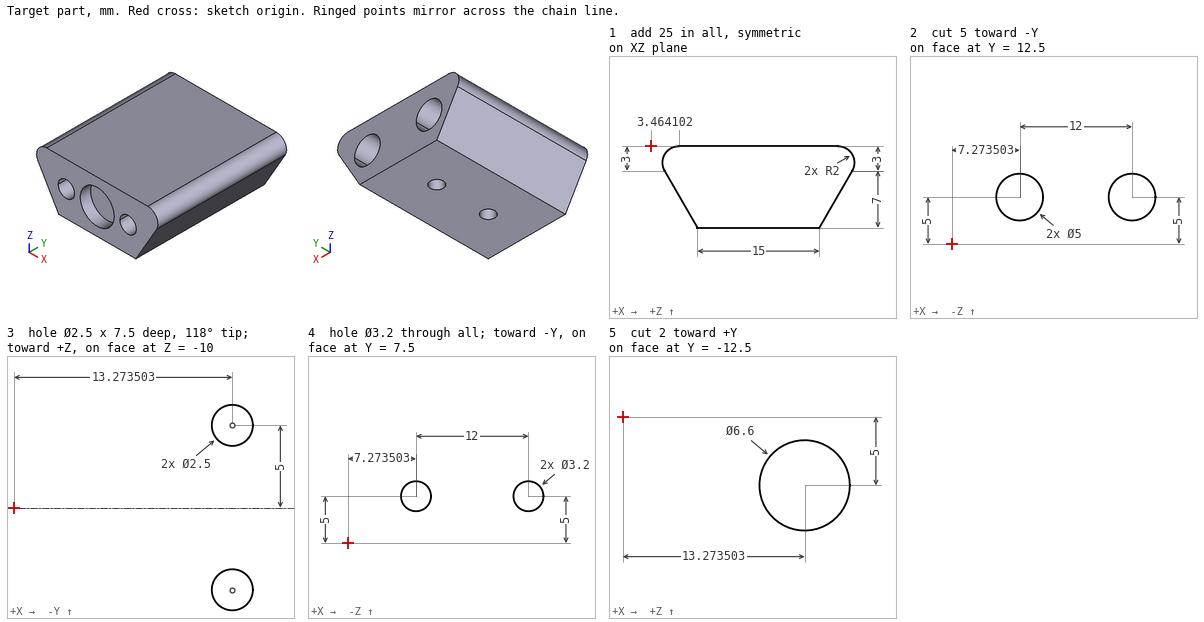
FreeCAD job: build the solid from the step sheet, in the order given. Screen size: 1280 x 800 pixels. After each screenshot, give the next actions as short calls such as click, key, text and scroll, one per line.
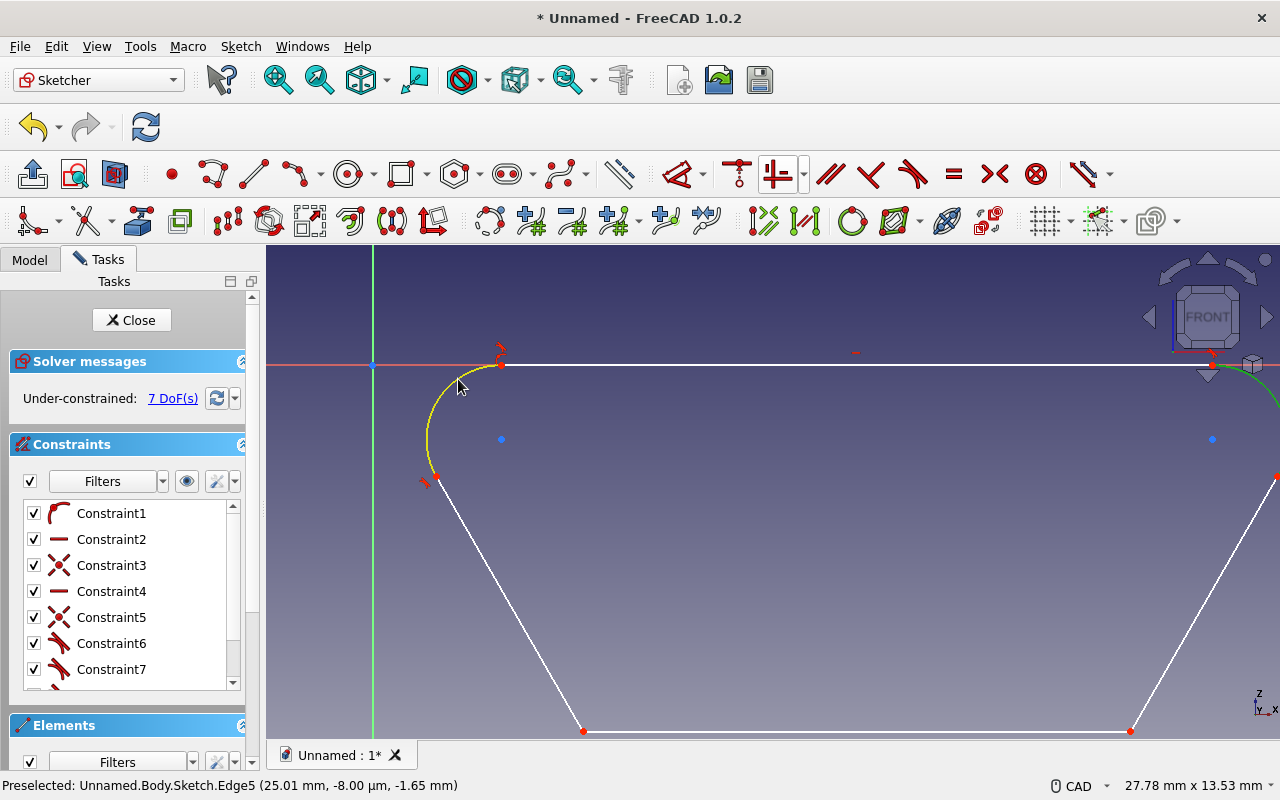
click(457, 379)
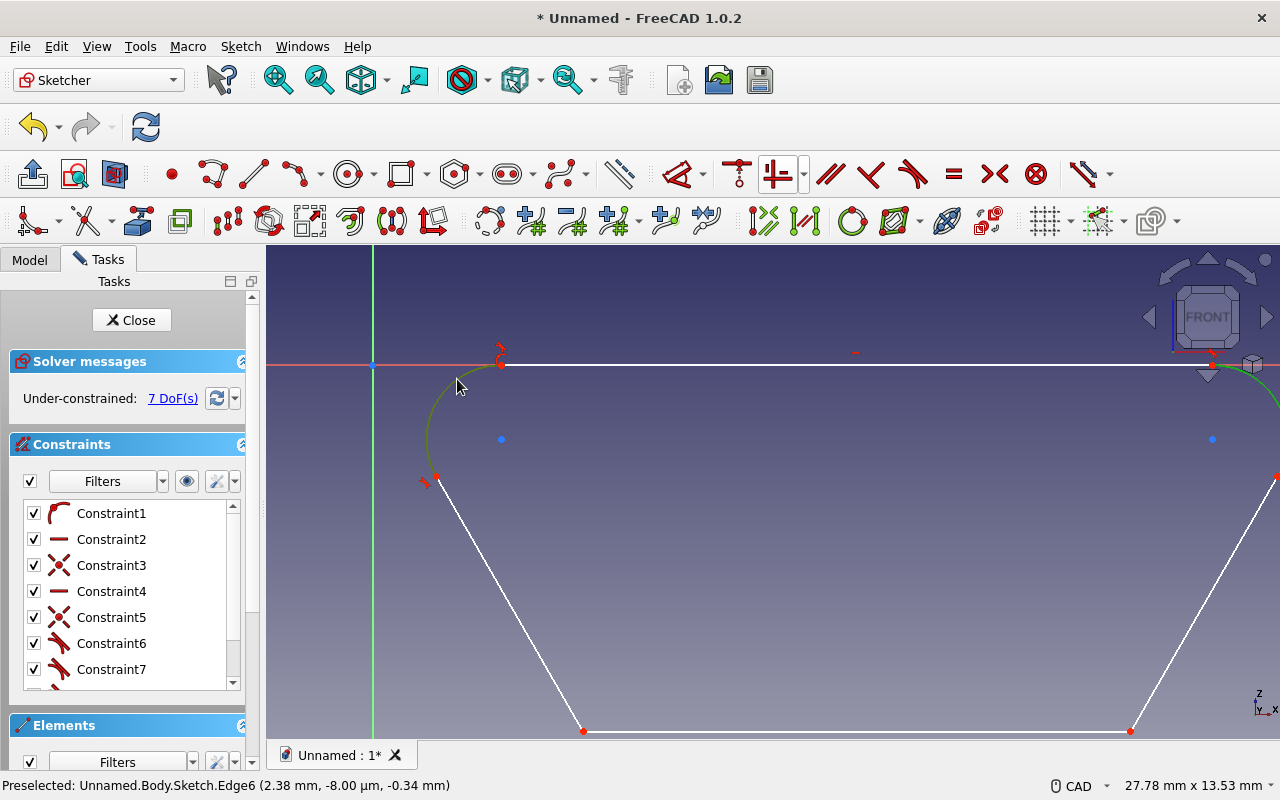
click(954, 174)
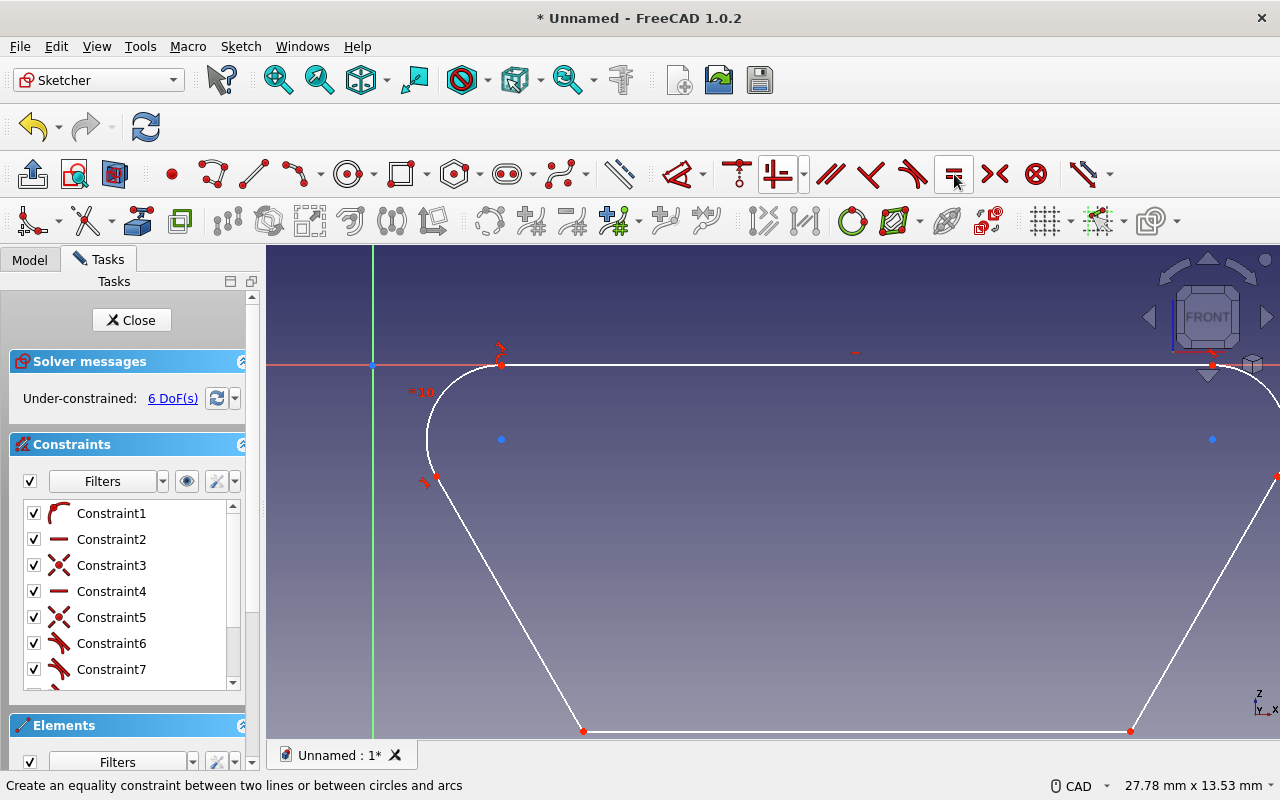
click(676, 174)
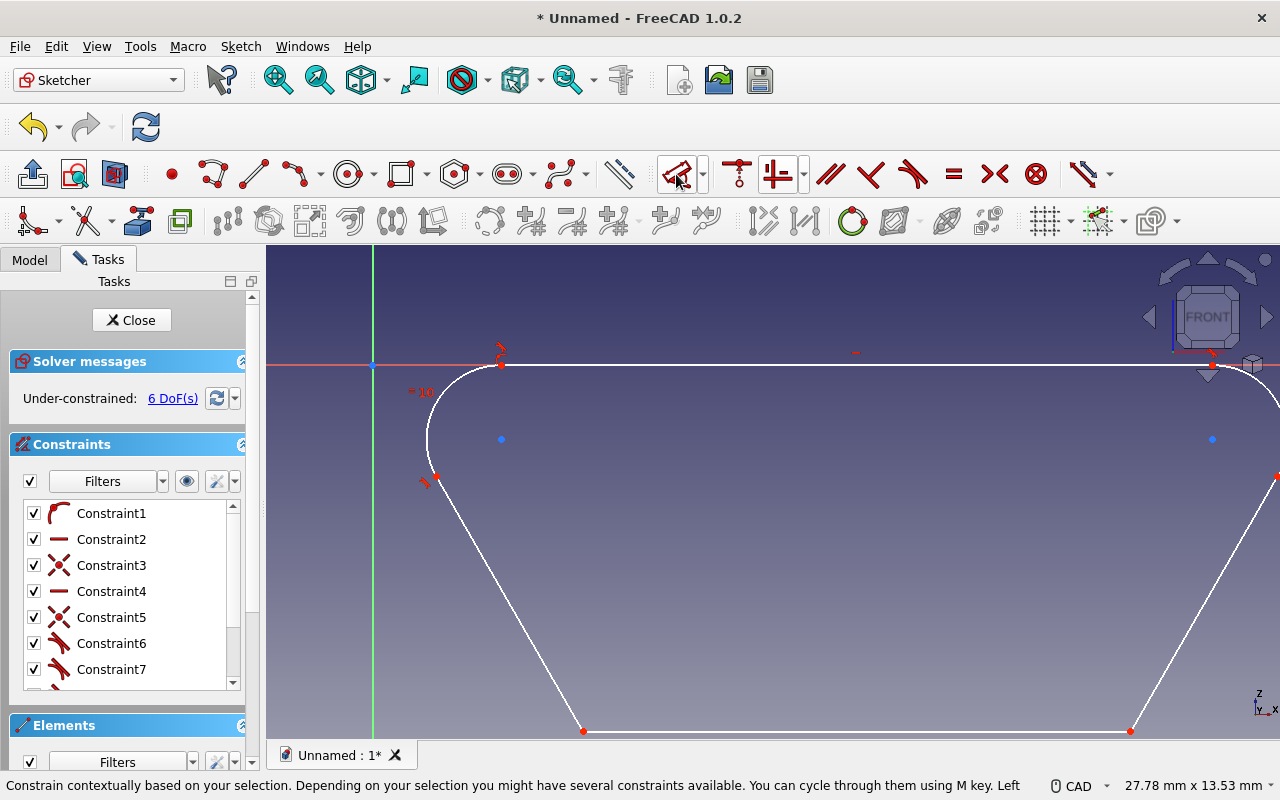
scroll(458, 379, down, 2)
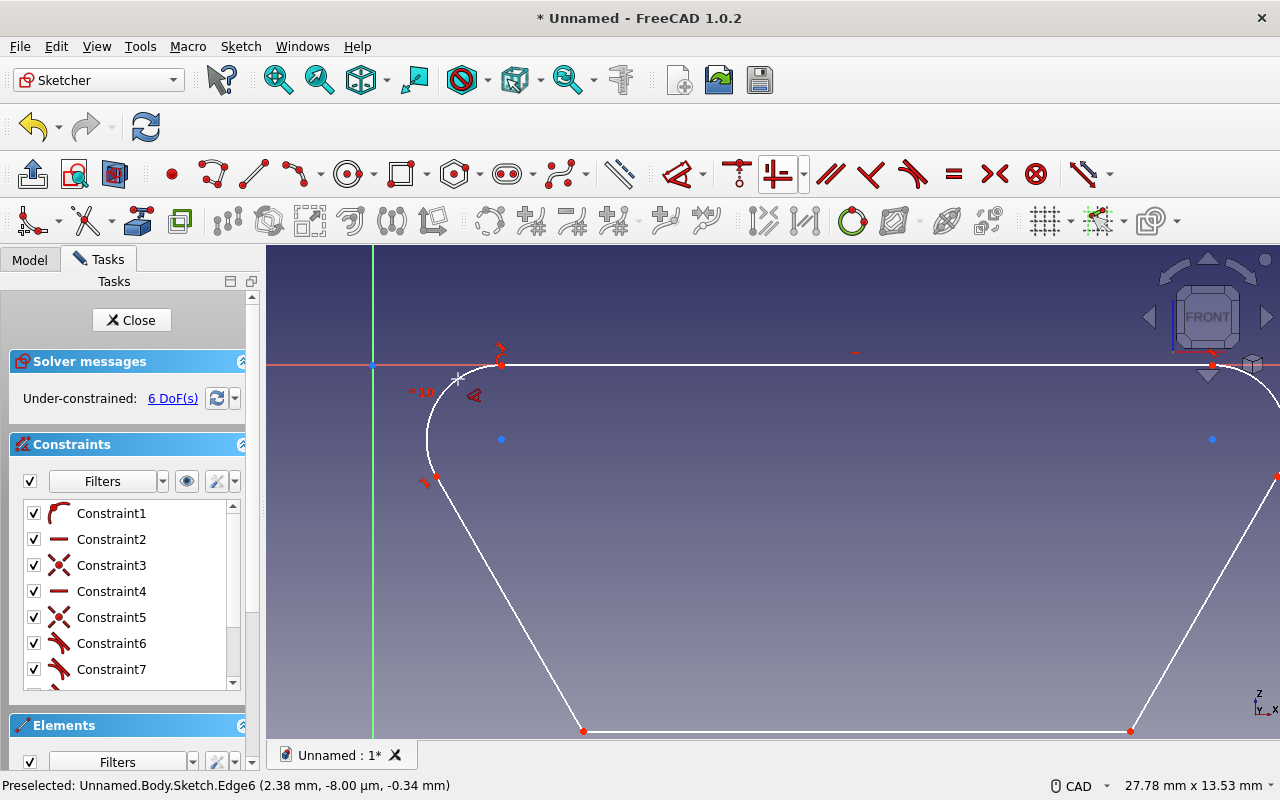
click(1014, 414)
click(1046, 410)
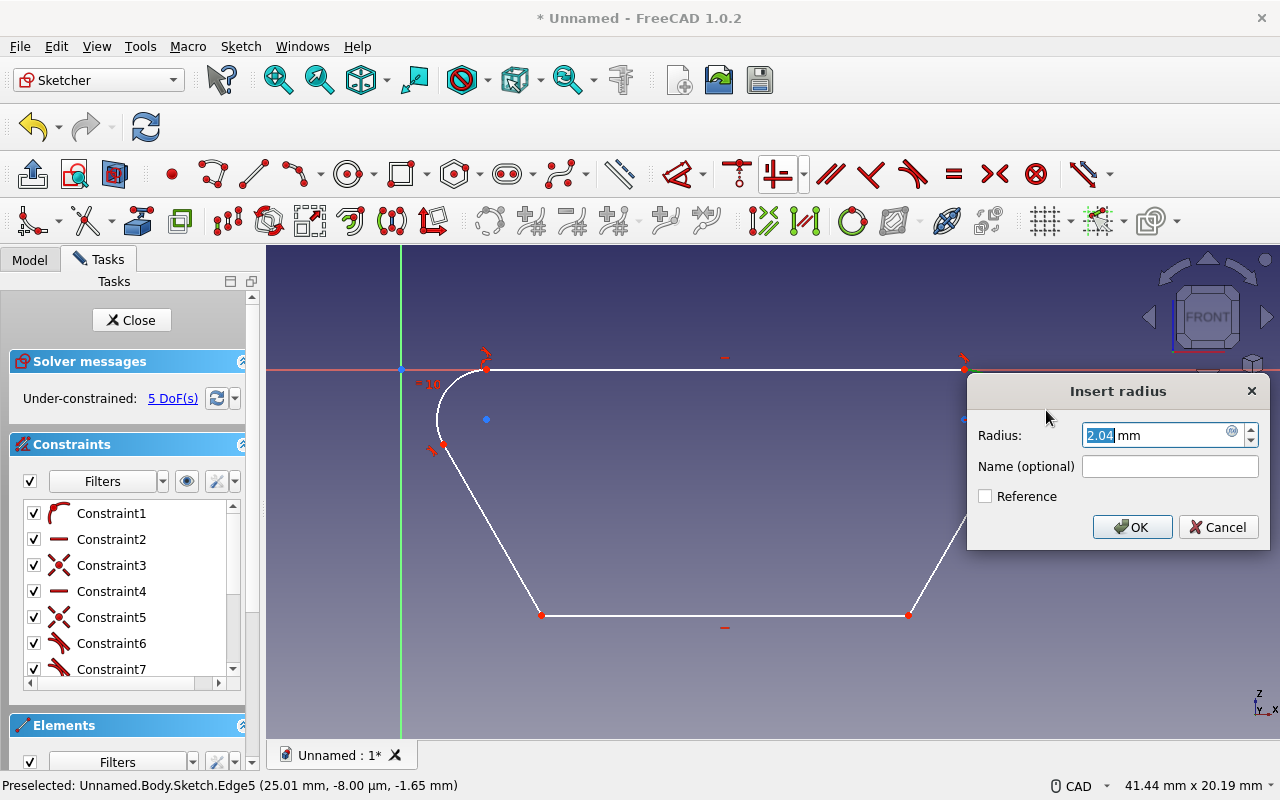
text(2)
key(Return)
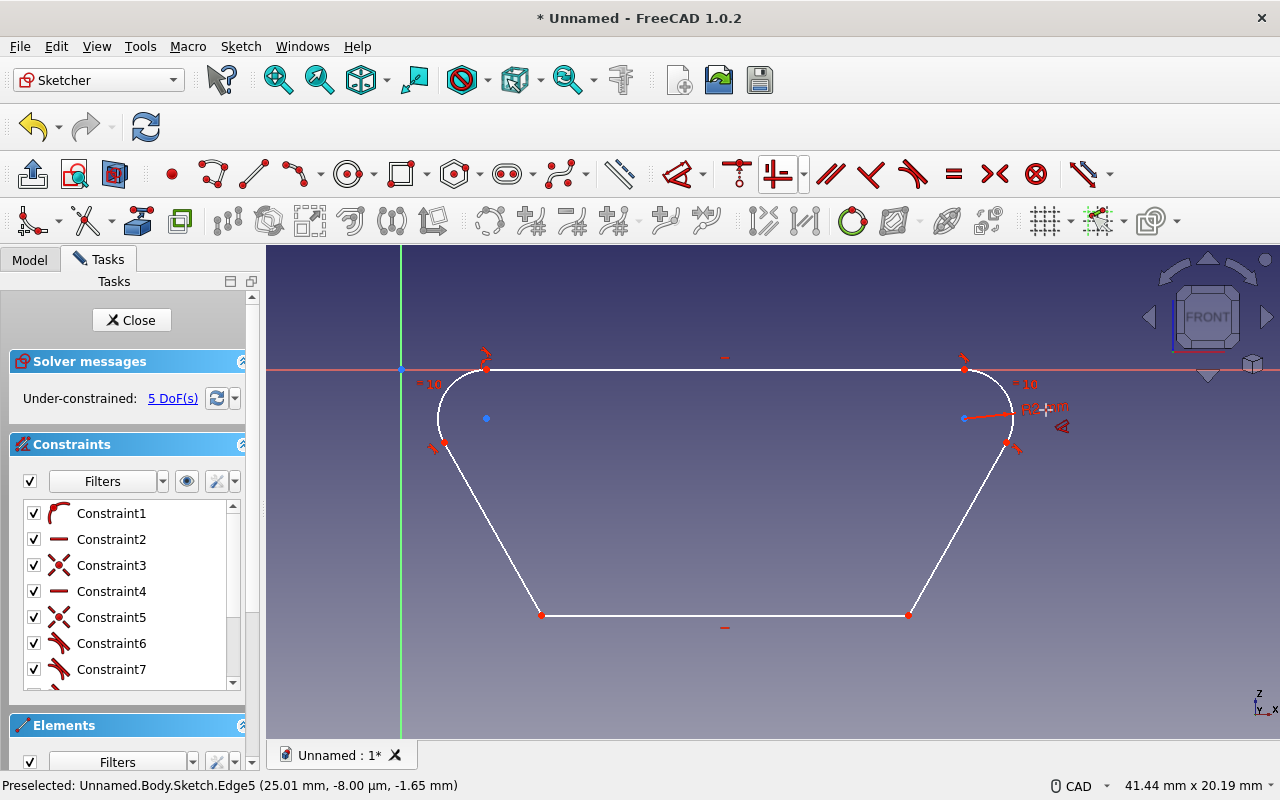
click(799, 616)
click(725, 650)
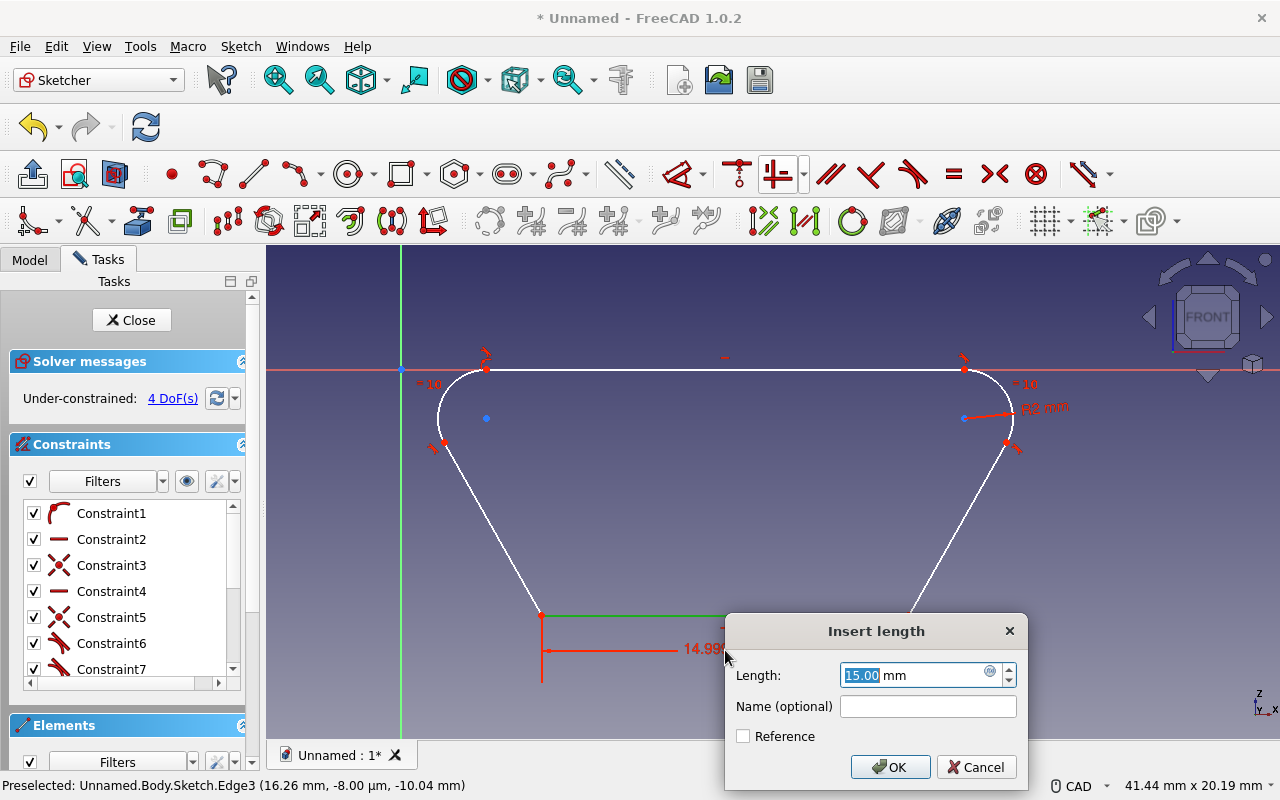
text(15)
key(Return)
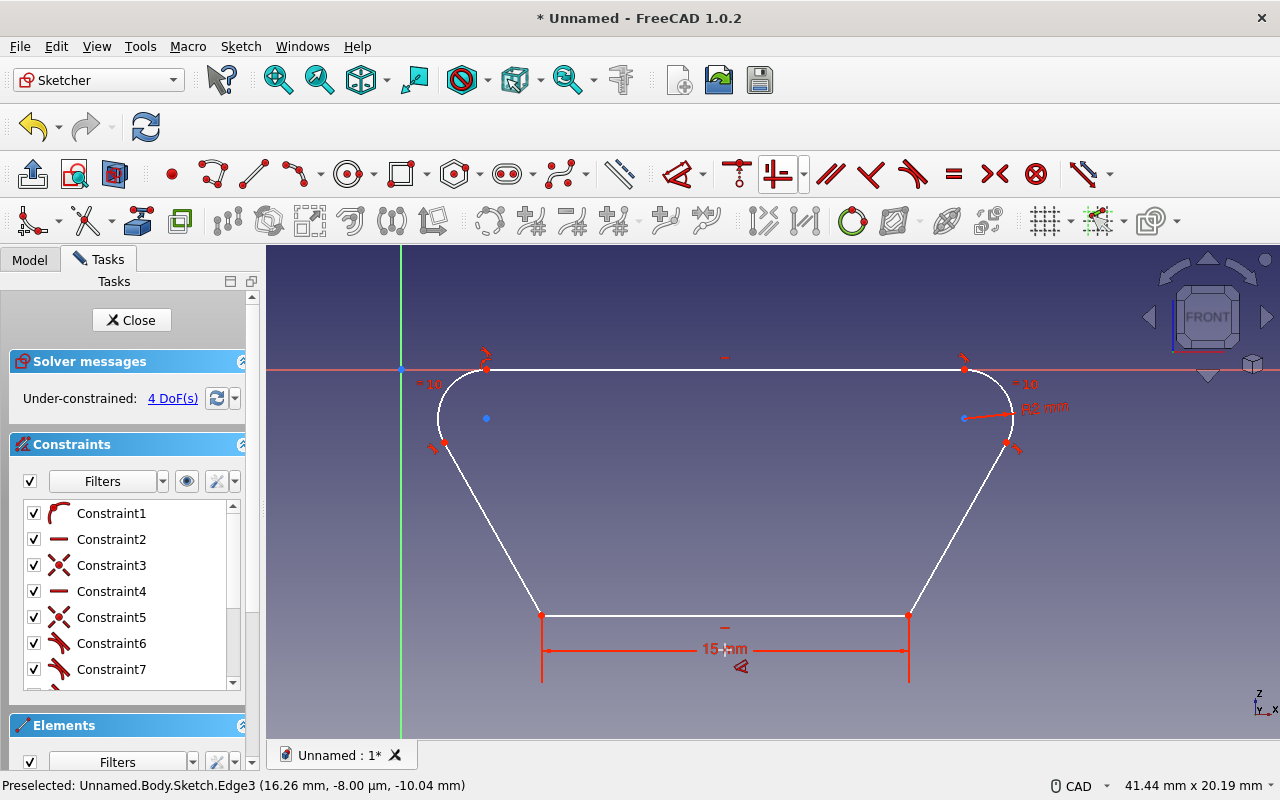
click(1007, 443)
click(367, 406)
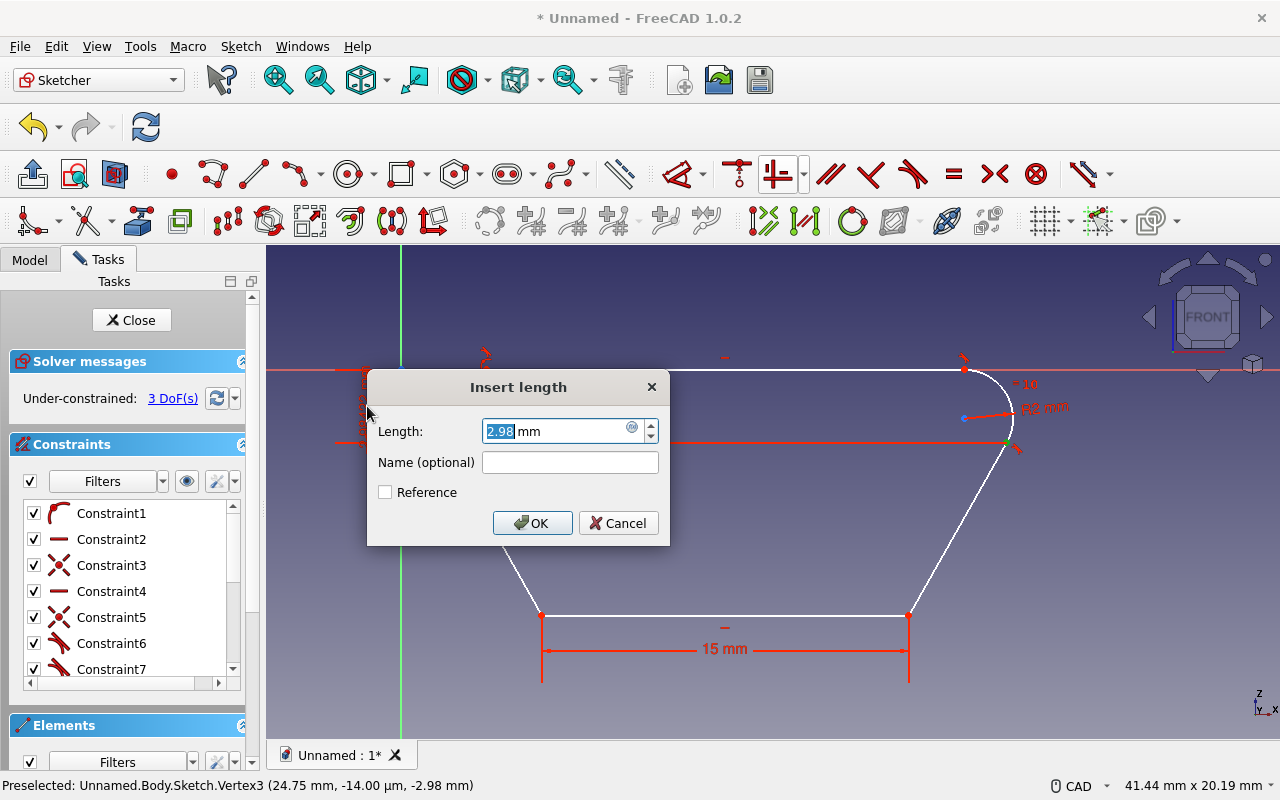
text(3)
key(Return)